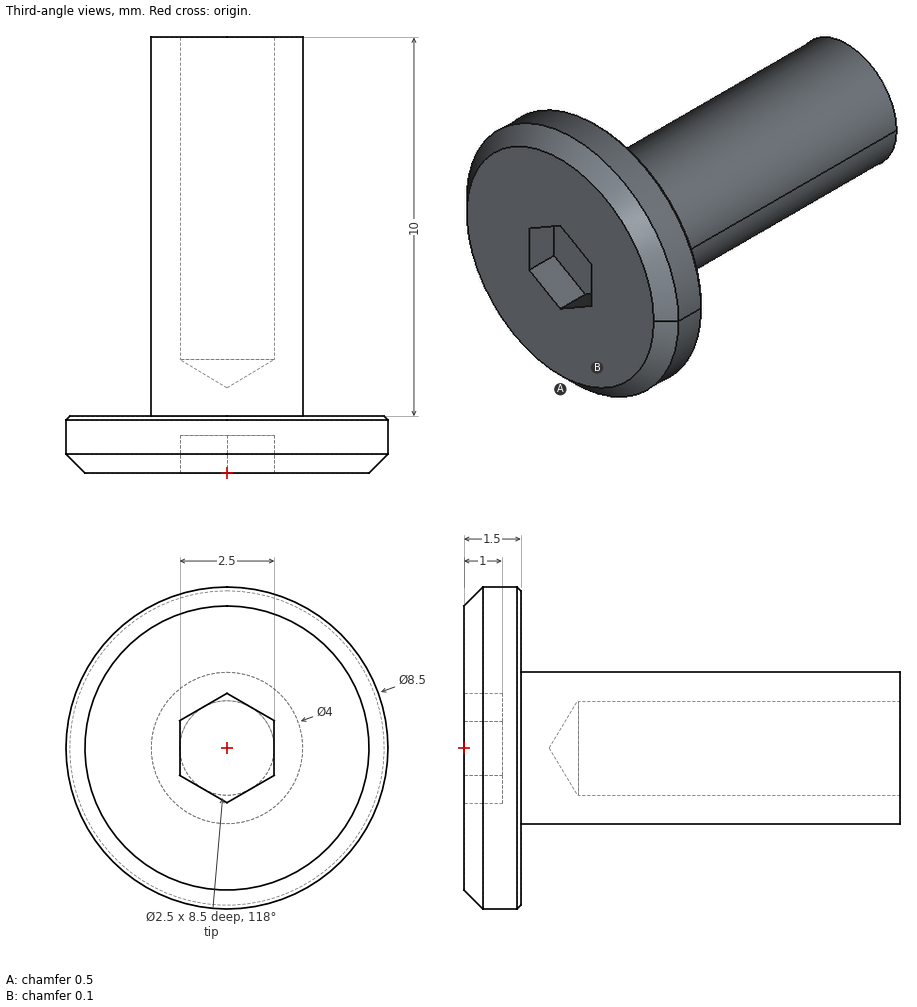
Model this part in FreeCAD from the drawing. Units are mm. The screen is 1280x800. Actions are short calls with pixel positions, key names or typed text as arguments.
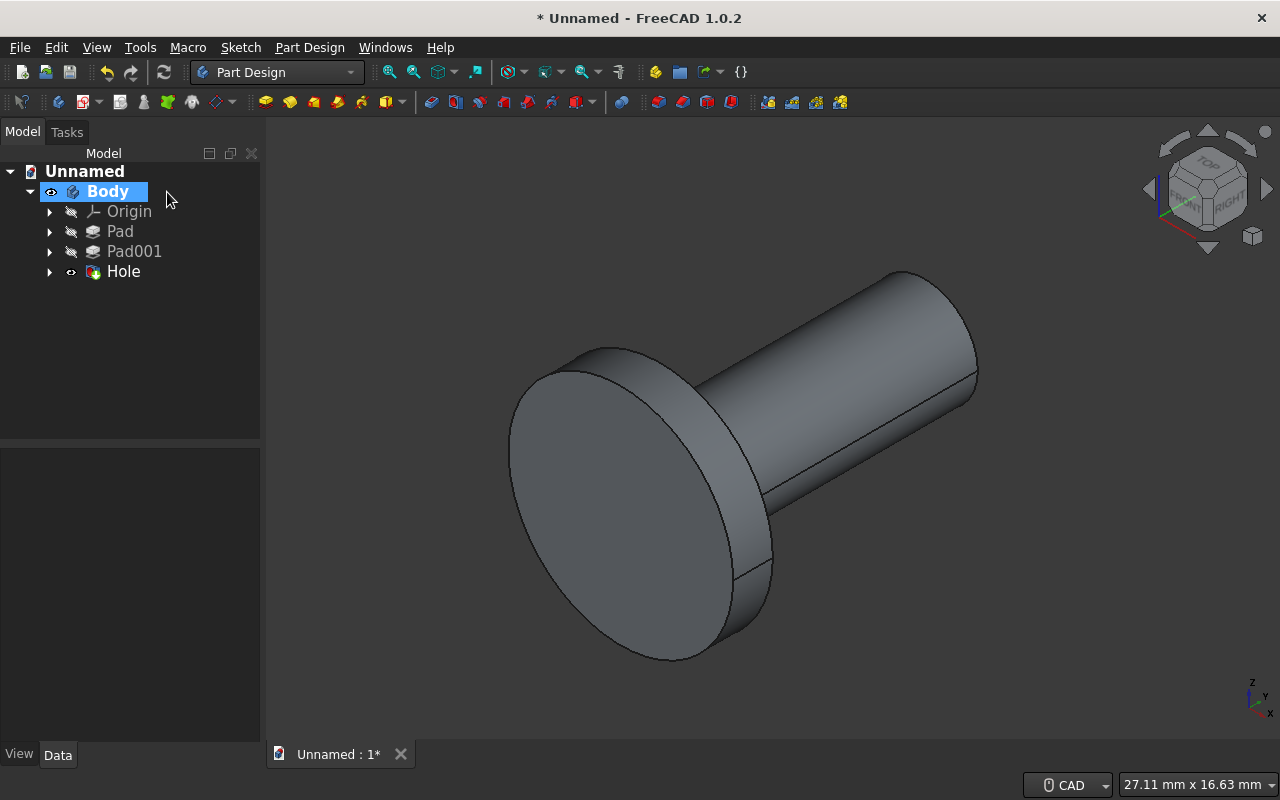
click(621, 515)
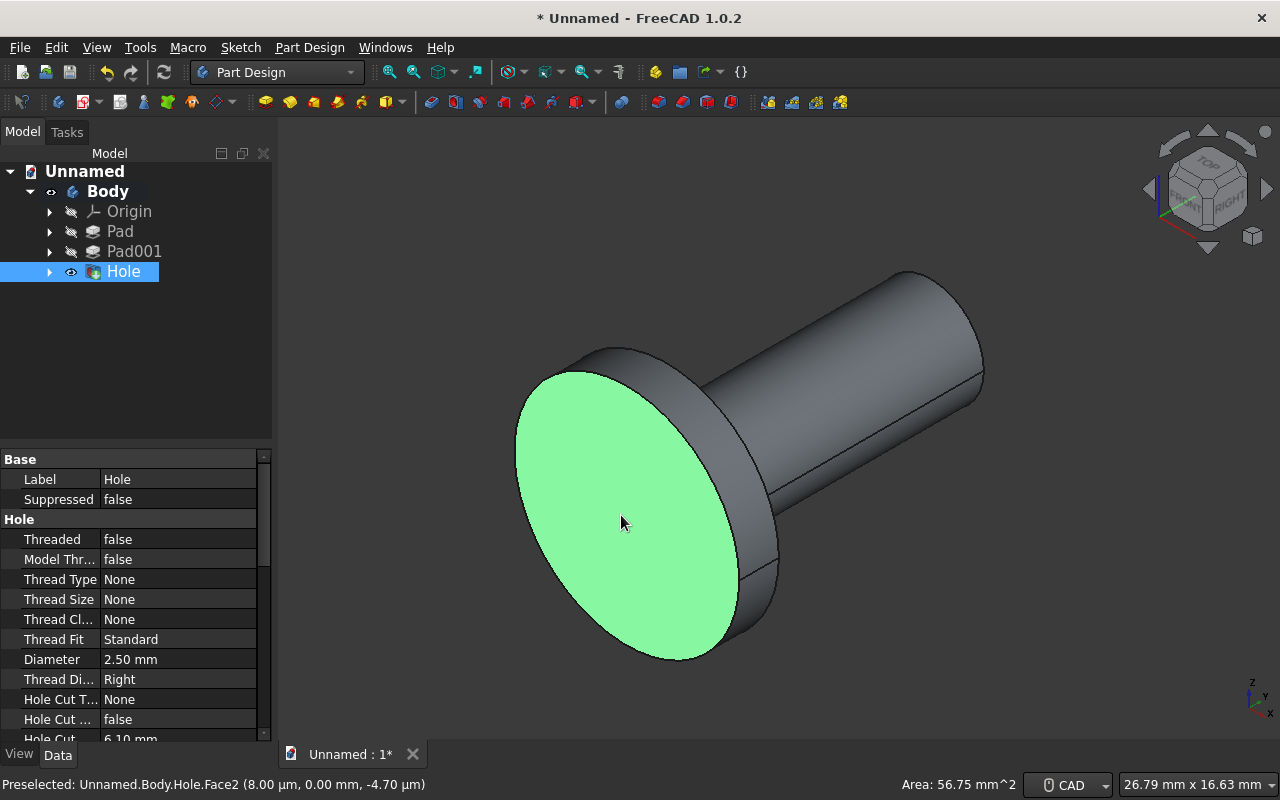
click(84, 102)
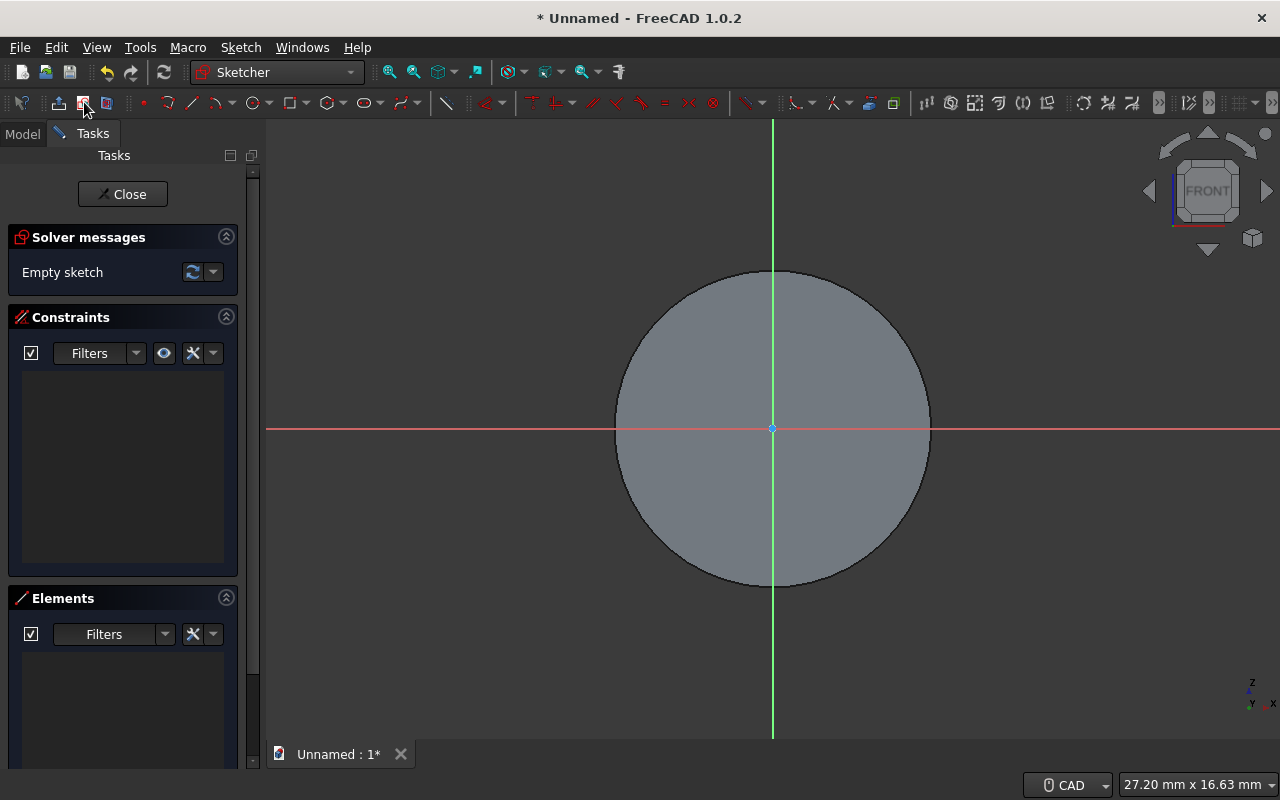
scroll(795, 429, up, 7)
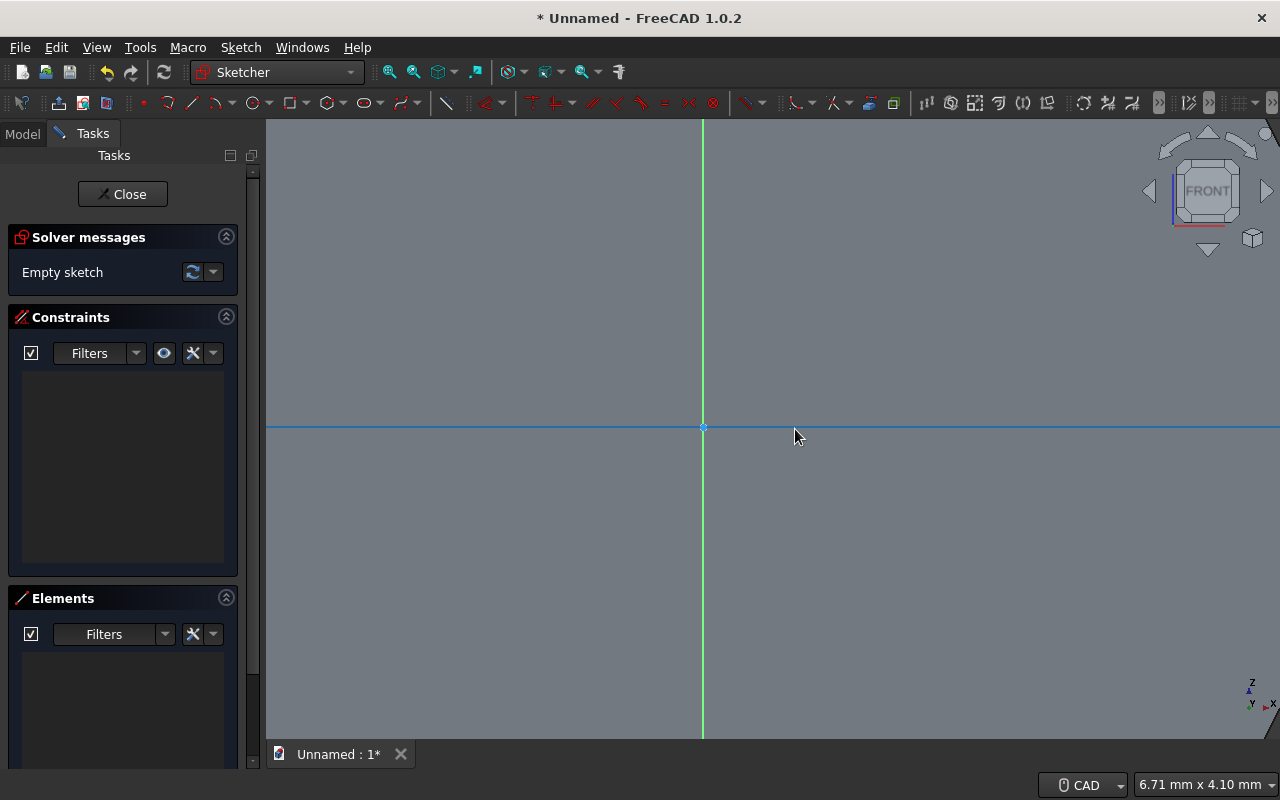
click(328, 104)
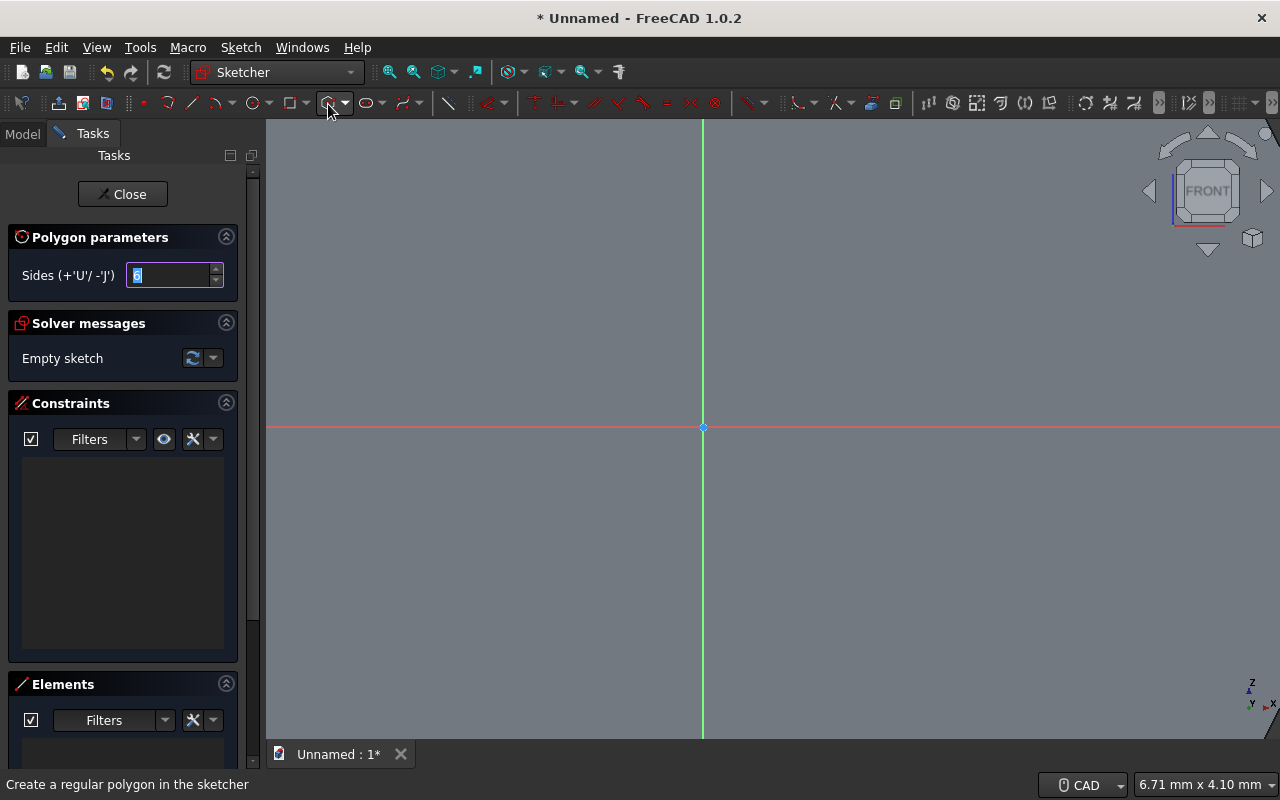
click(703, 427)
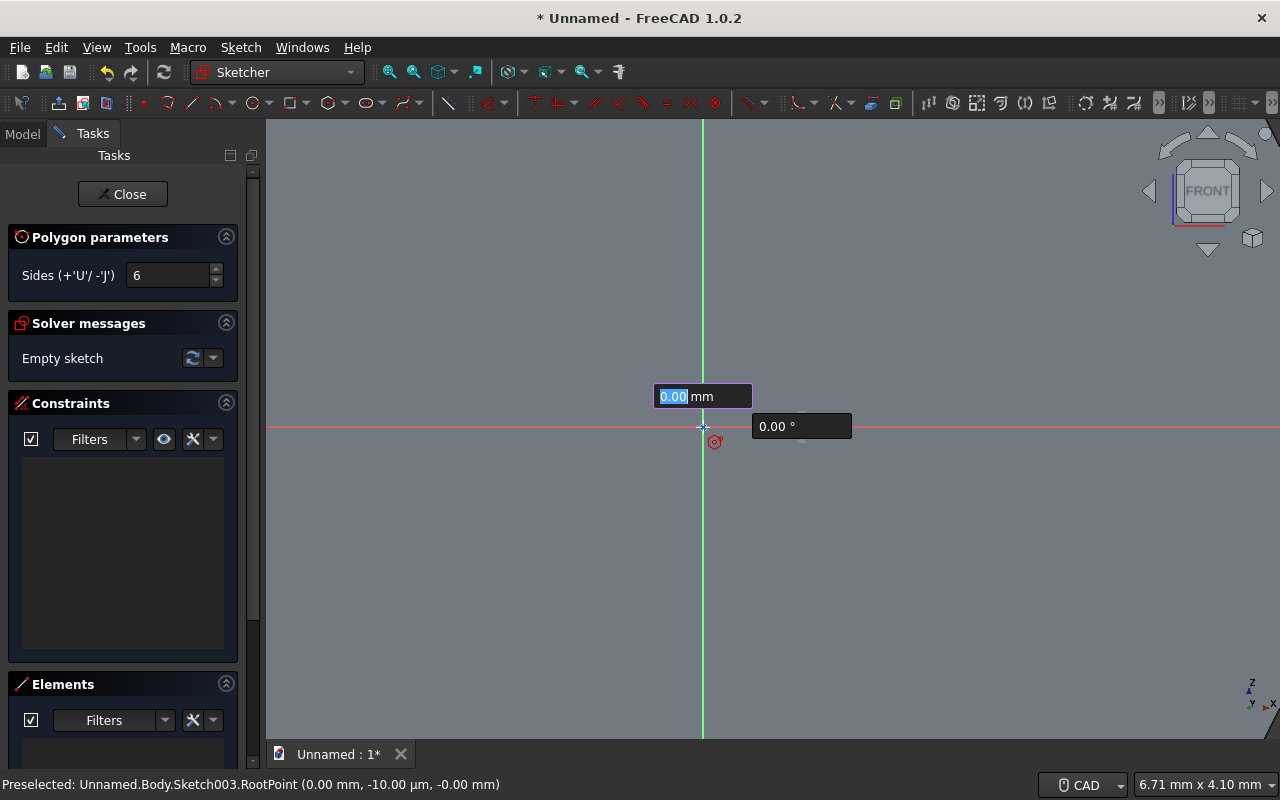
click(703, 209)
right_click(703, 209)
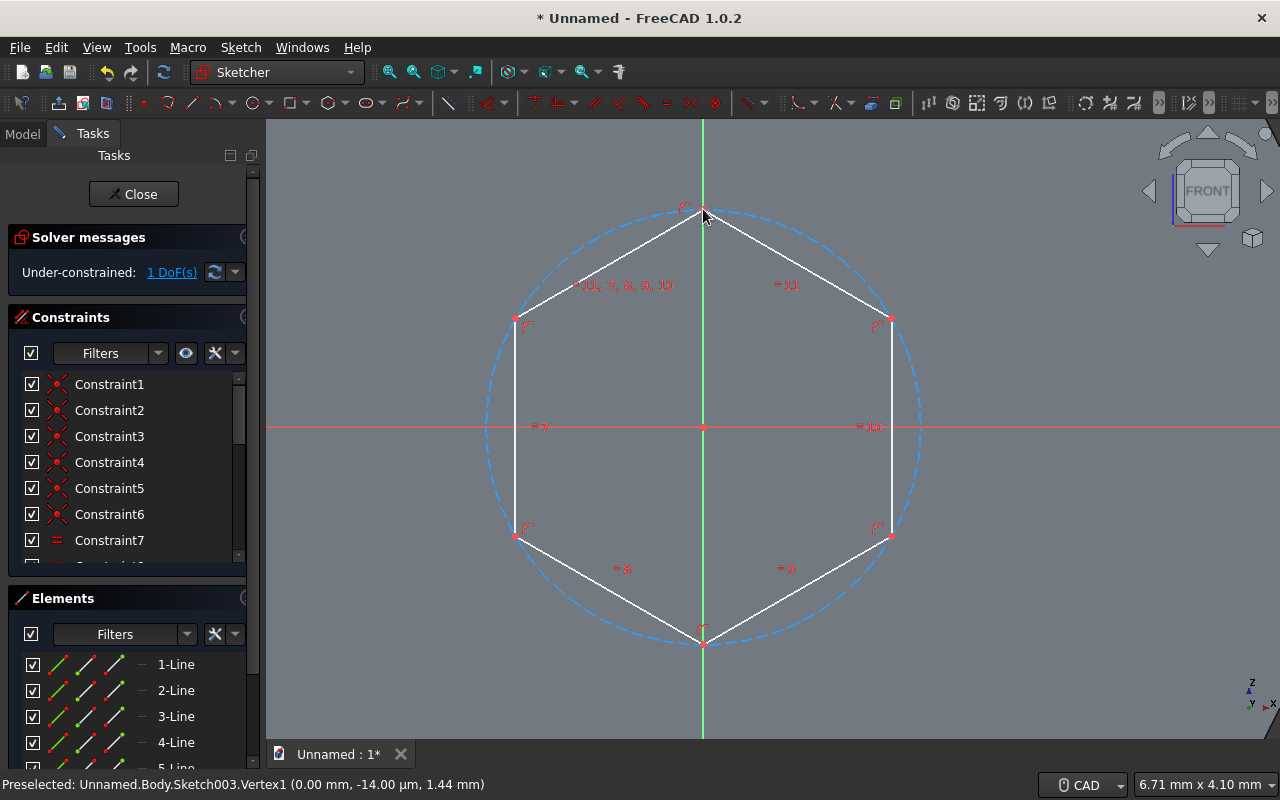
click(515, 319)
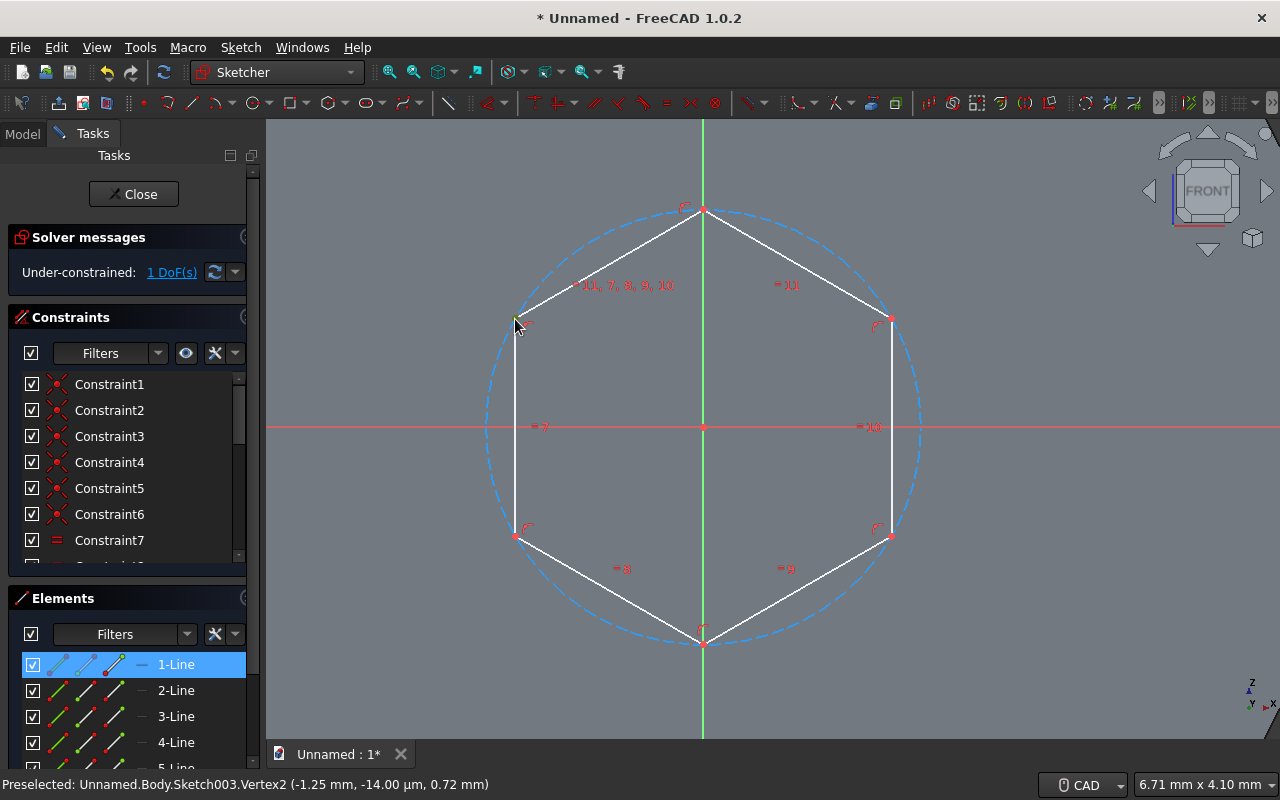
click(892, 536)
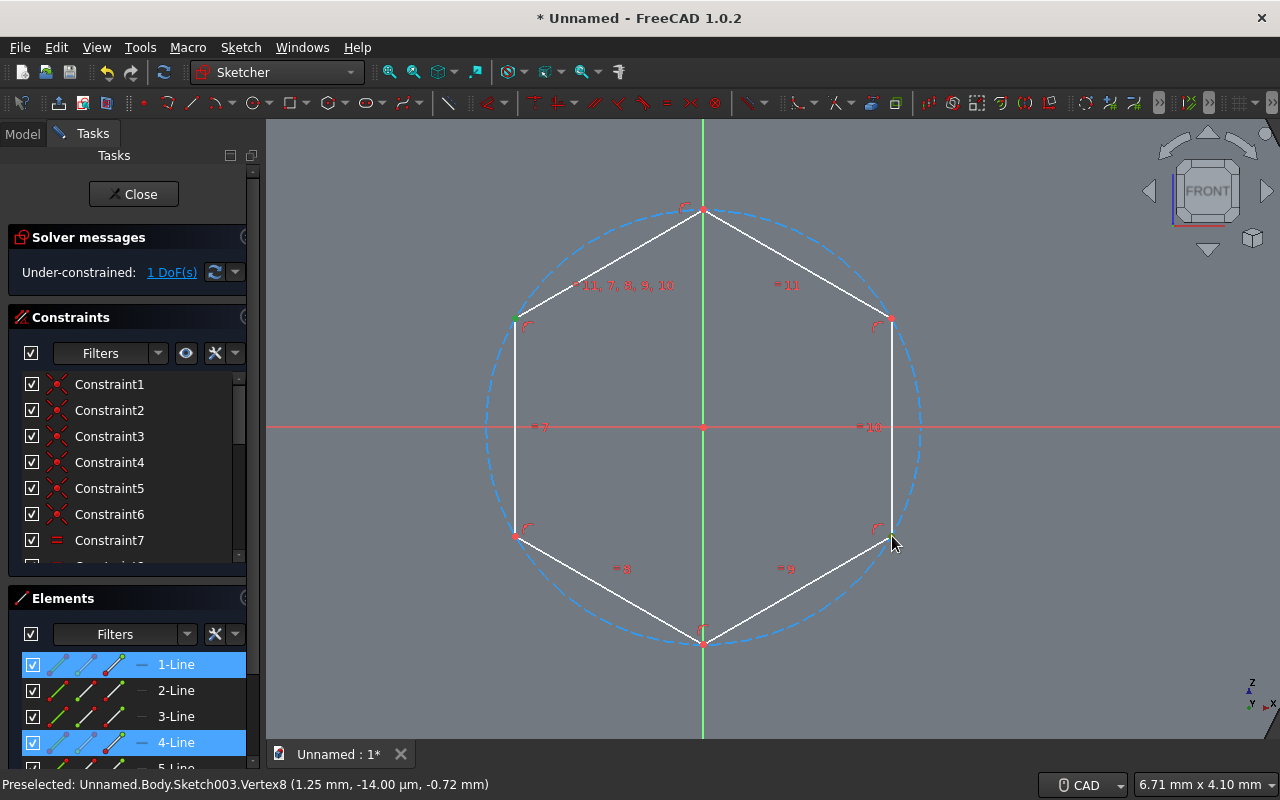
click(506, 104)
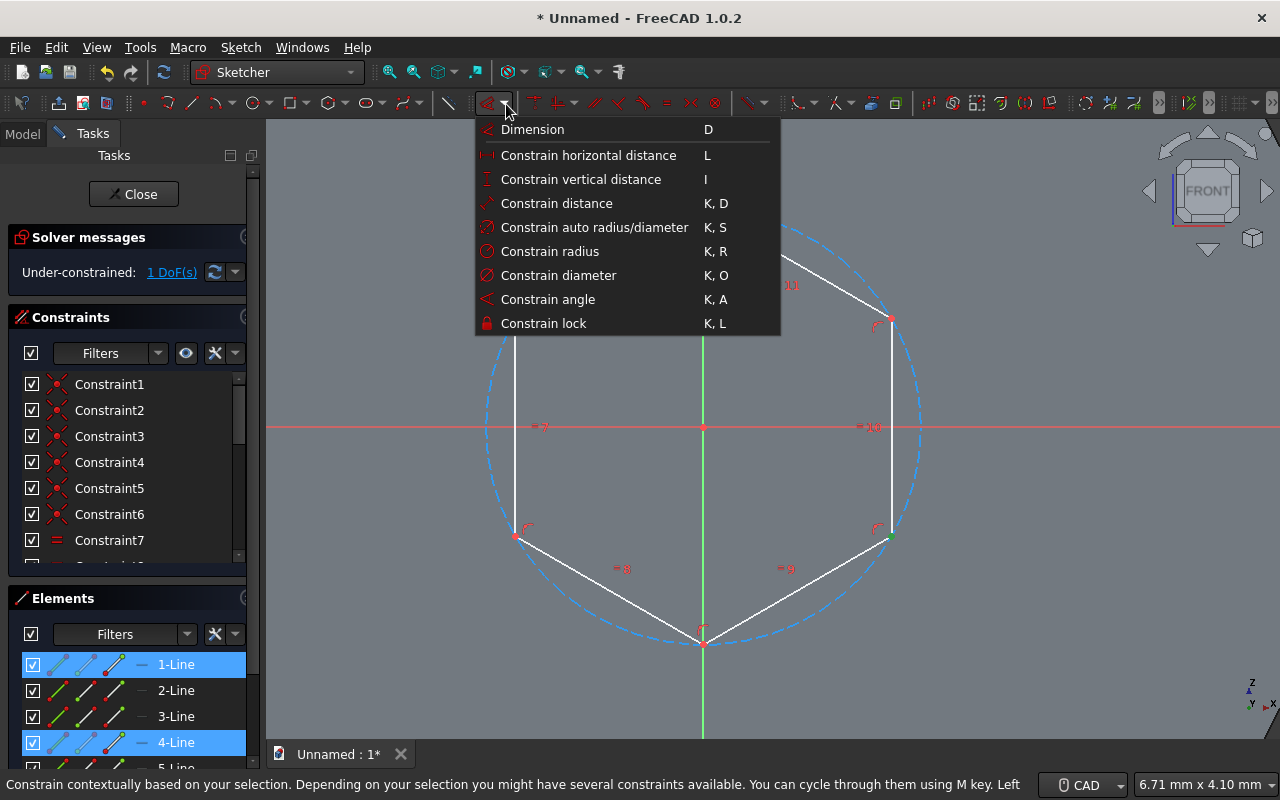
click(628, 155)